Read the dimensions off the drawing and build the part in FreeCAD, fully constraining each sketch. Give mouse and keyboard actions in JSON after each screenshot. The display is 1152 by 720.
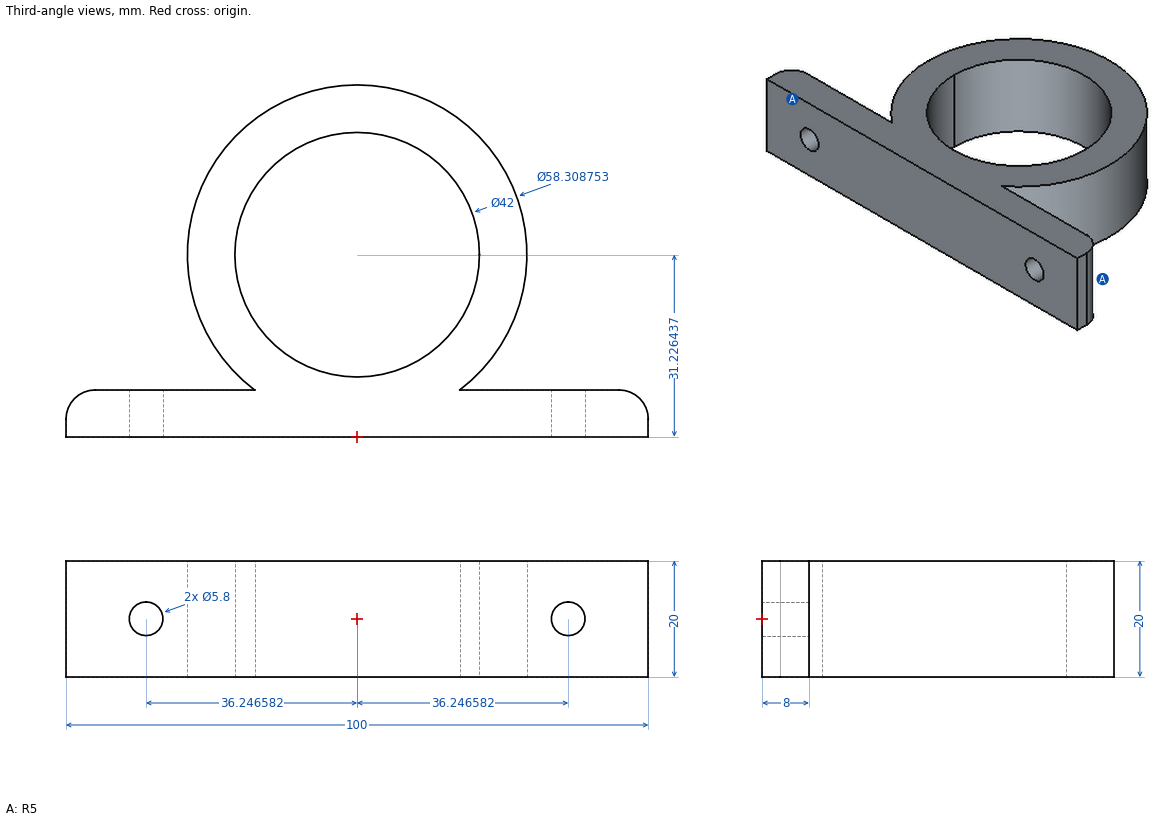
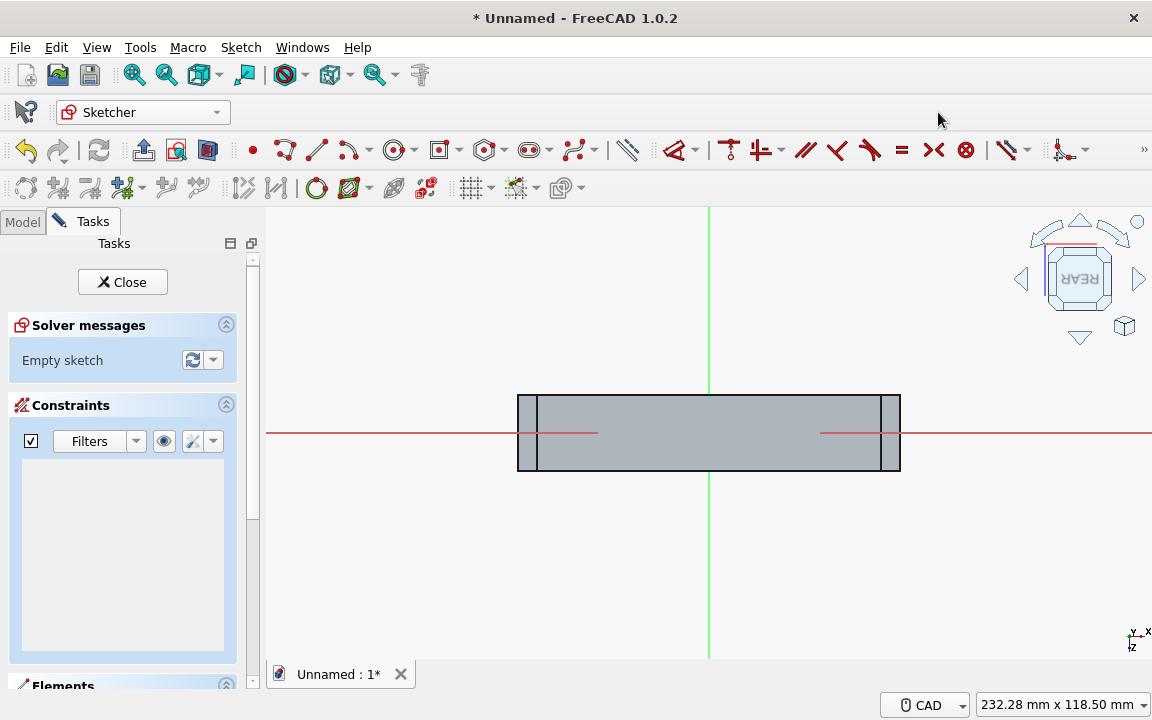
{"action": "scroll", "coordinate": [848, 433], "scroll_direction": "up", "scroll_amount": 2}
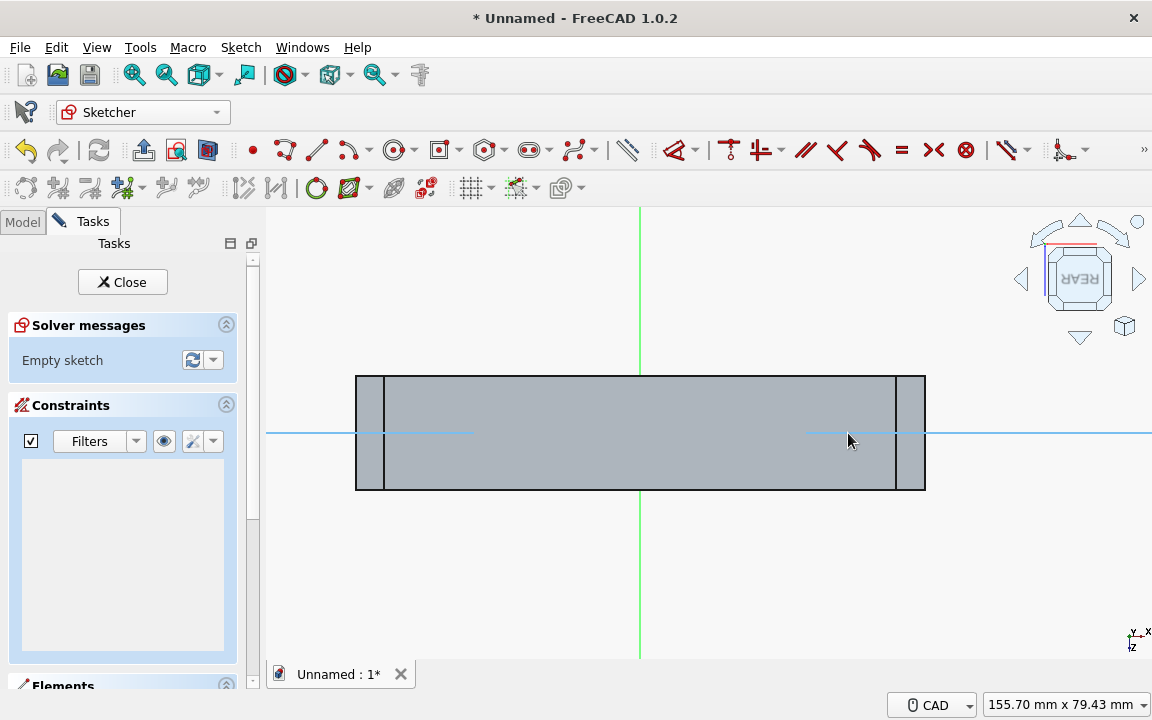
{"action": "left_click", "coordinate": [394, 150]}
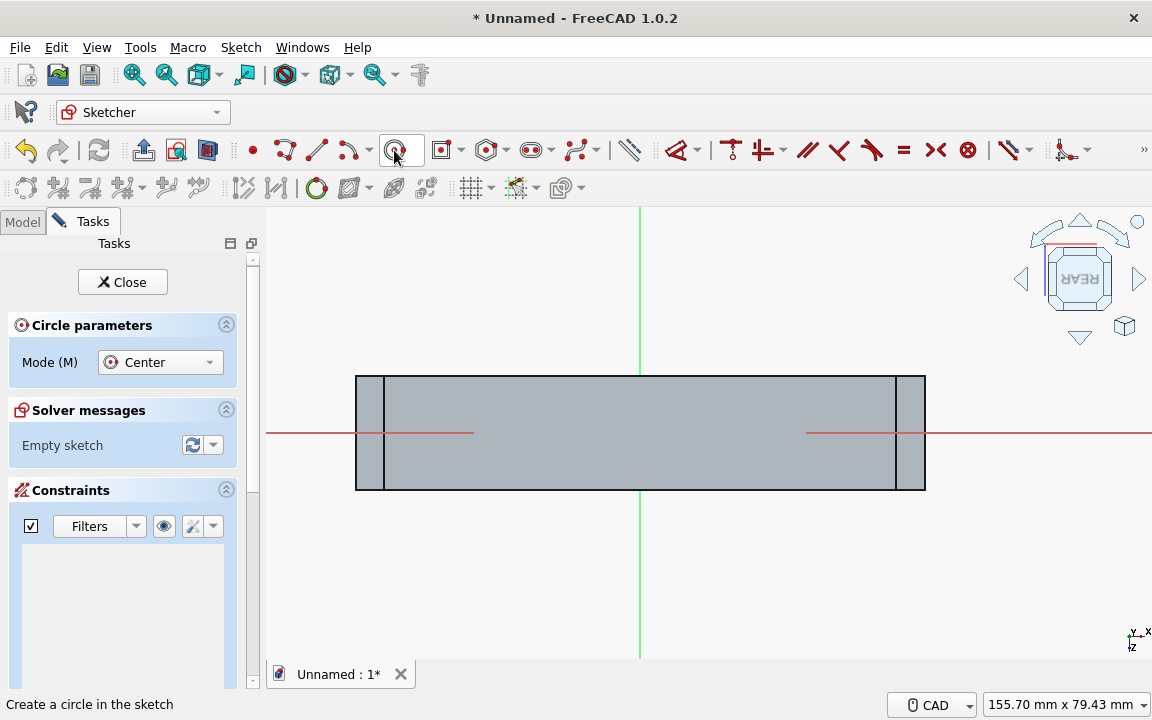
{"action": "scroll", "coordinate": [434, 433], "scroll_direction": "up", "scroll_amount": 2}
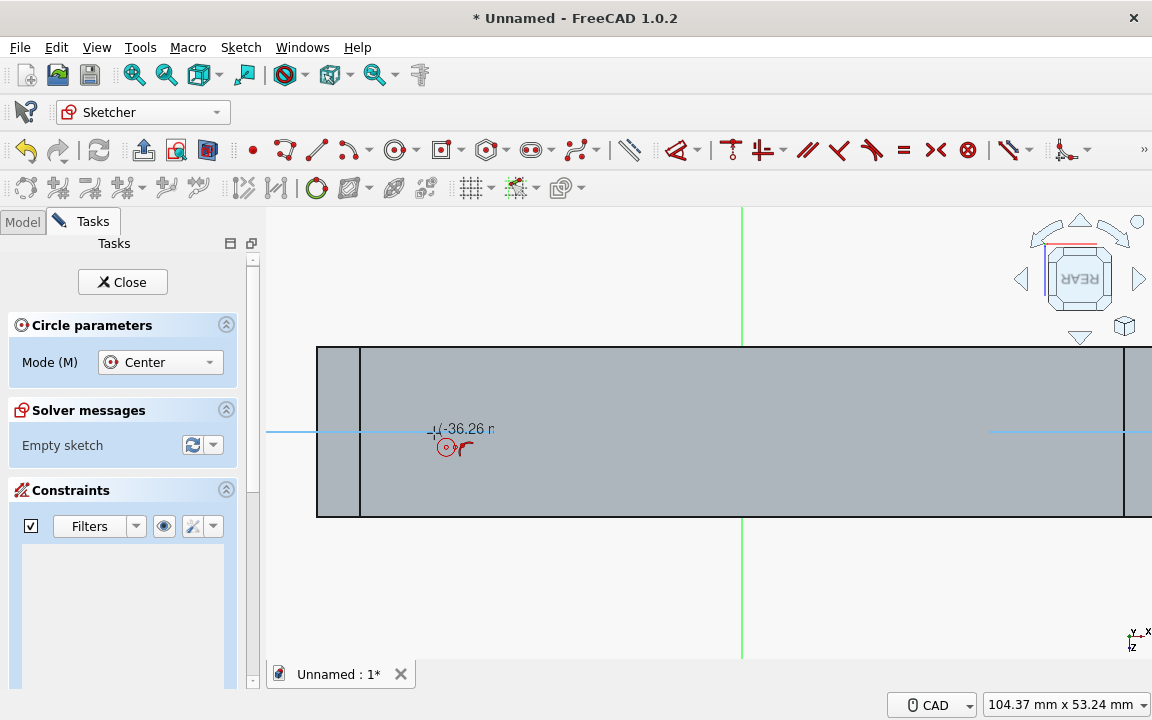
{"action": "left_click", "coordinate": [434, 432]}
{"action": "left_click", "coordinate": [451, 415]}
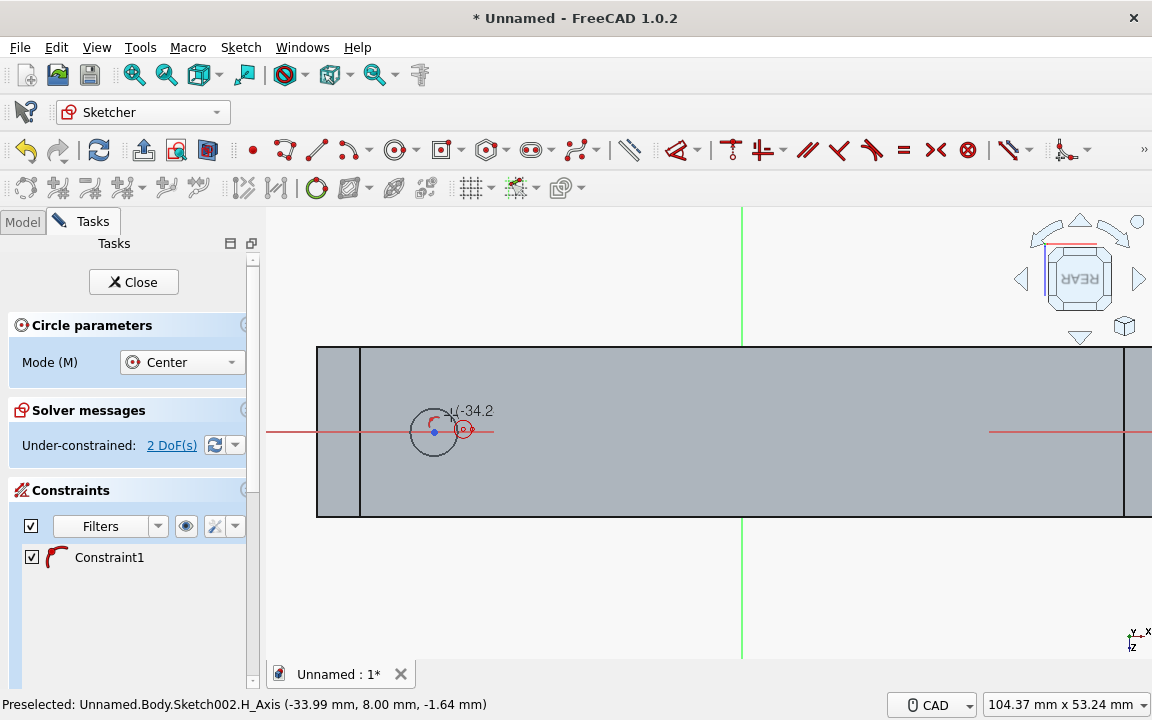
{"action": "scroll", "coordinate": [435, 434], "scroll_direction": "down", "scroll_amount": 2}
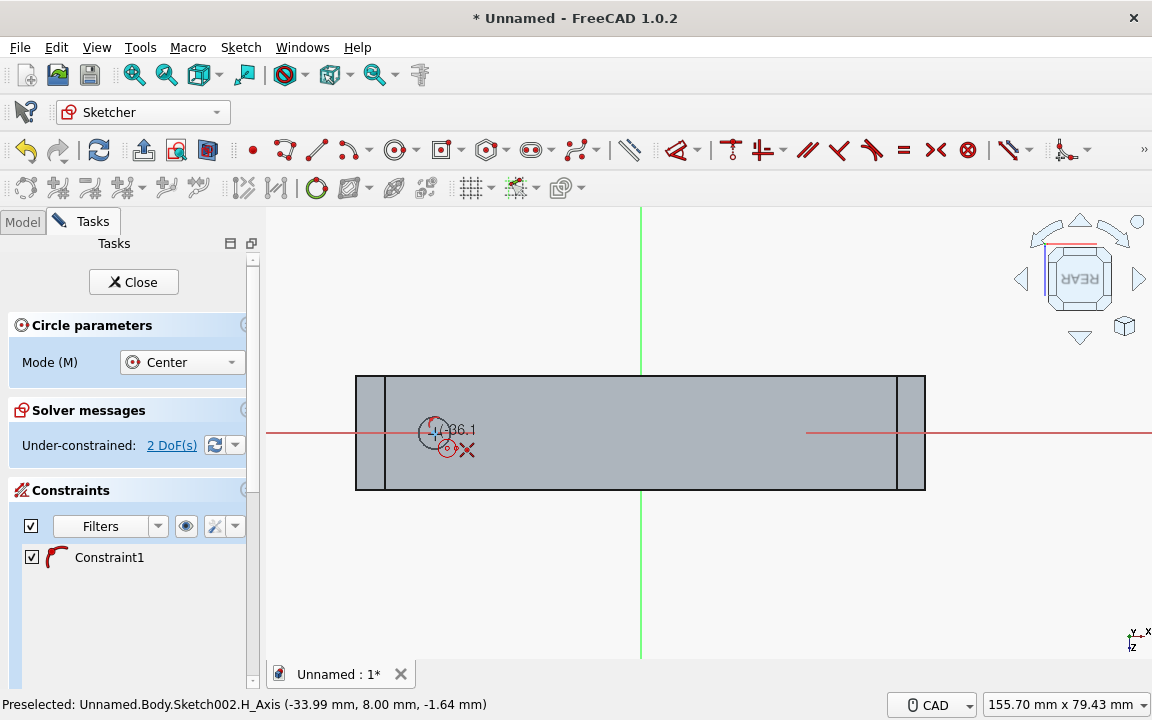
{"action": "scroll", "coordinate": [847, 433], "scroll_direction": "up", "scroll_amount": 2}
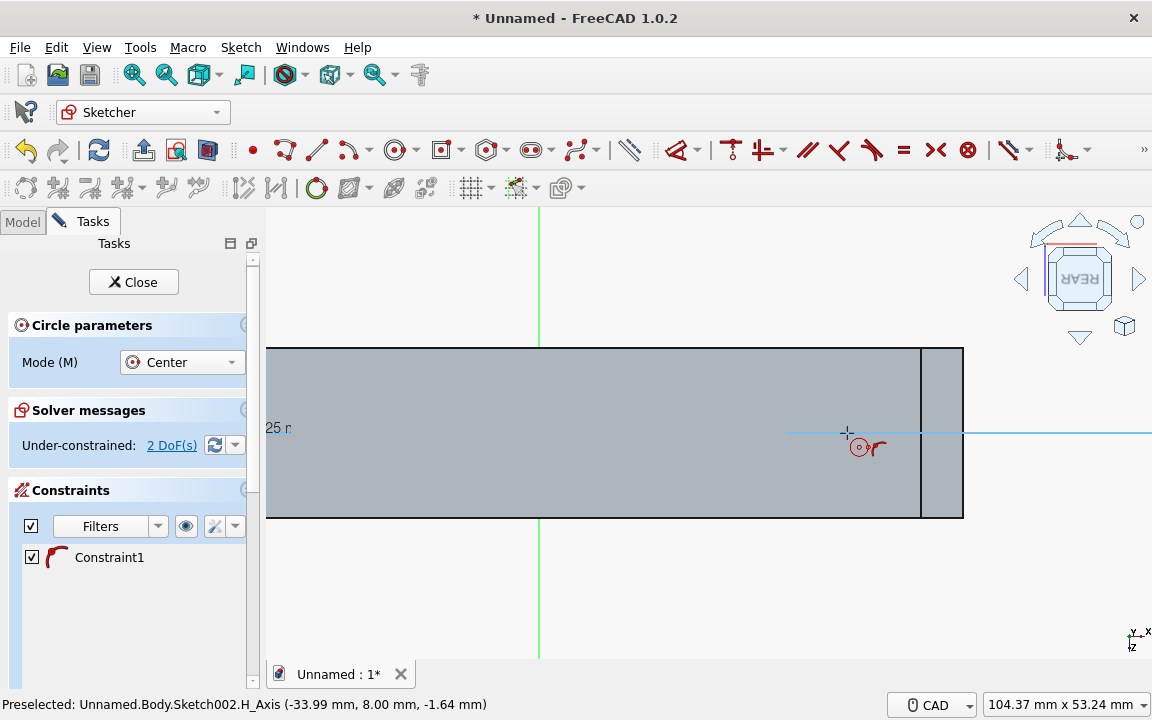
{"action": "left_click", "coordinate": [847, 433]}
{"action": "left_click", "coordinate": [864, 415]}
{"action": "key", "text": "Escape"}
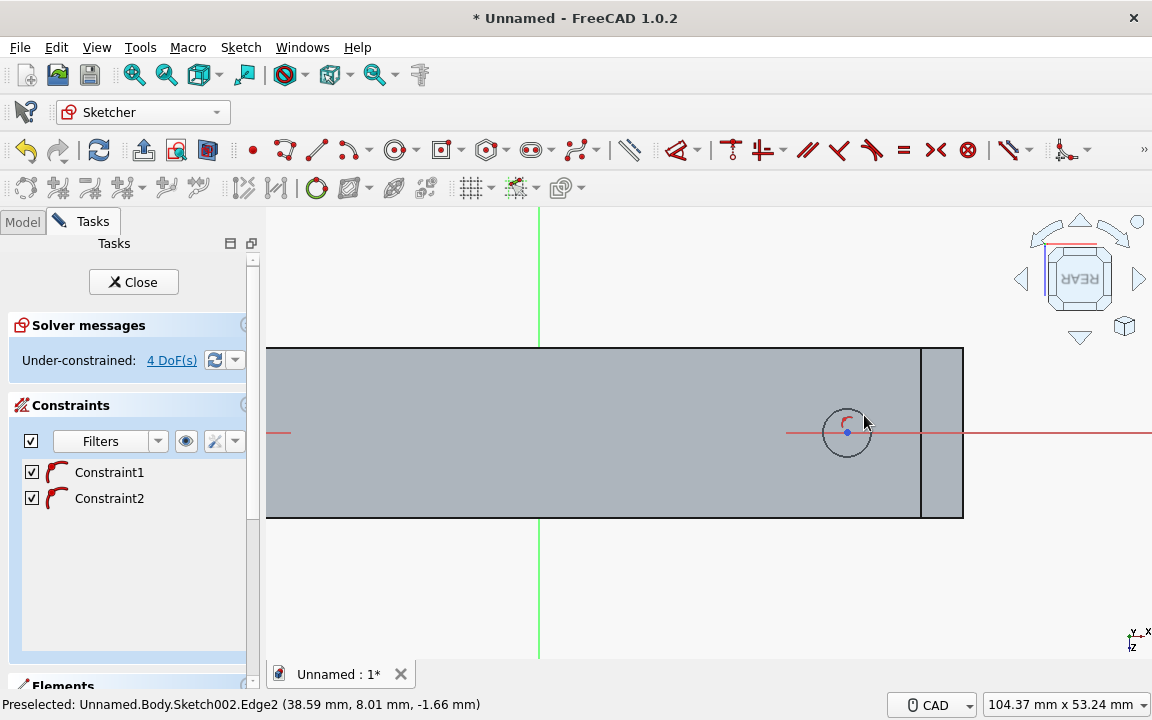
{"action": "scroll", "coordinate": [847, 433], "scroll_direction": "down", "scroll_amount": 2}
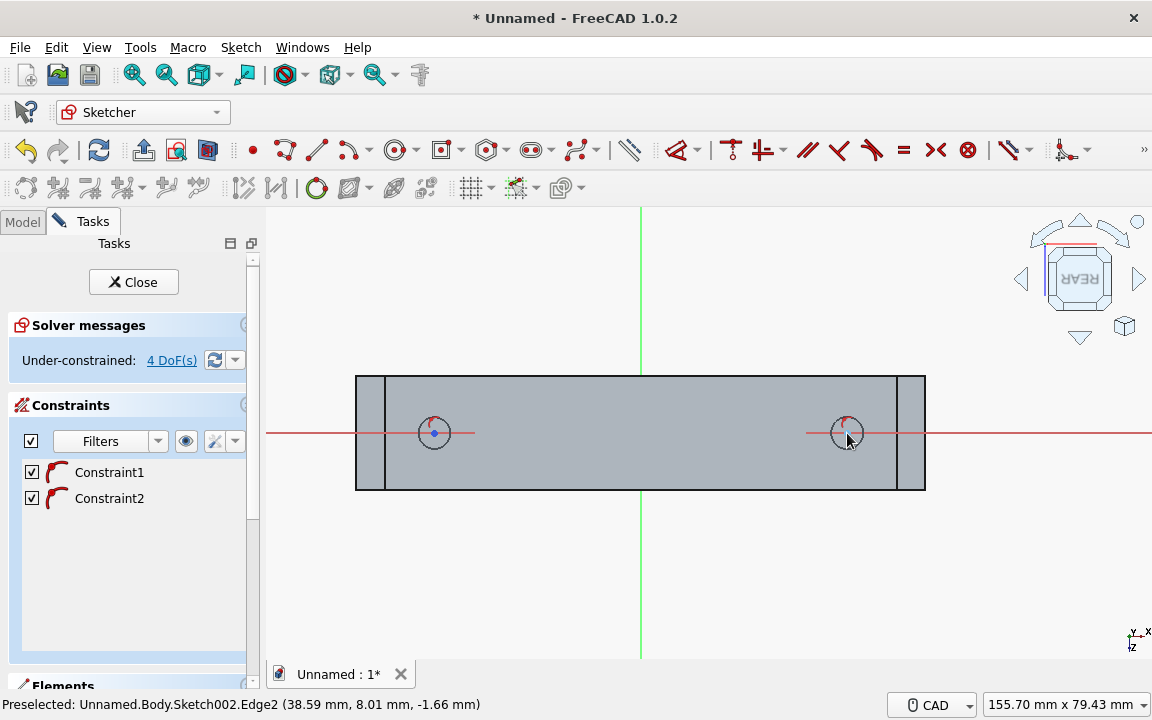
{"action": "scroll", "coordinate": [446, 422], "scroll_direction": "up", "scroll_amount": 2}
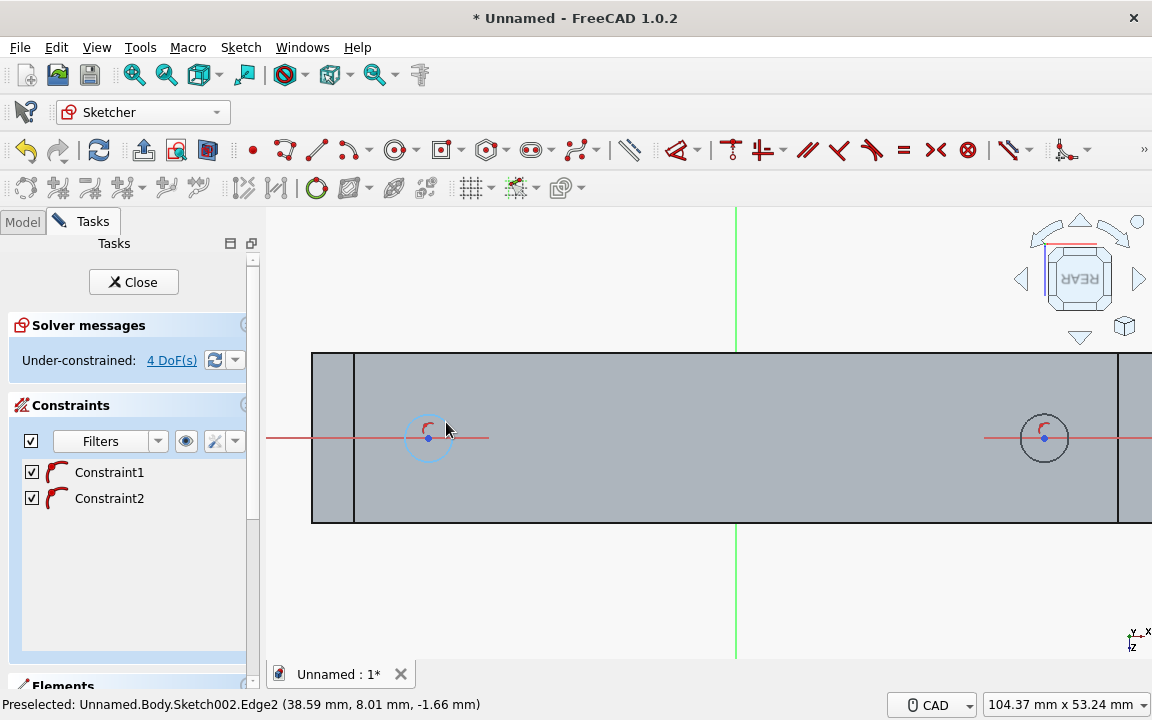
{"action": "left_click", "coordinate": [445, 422]}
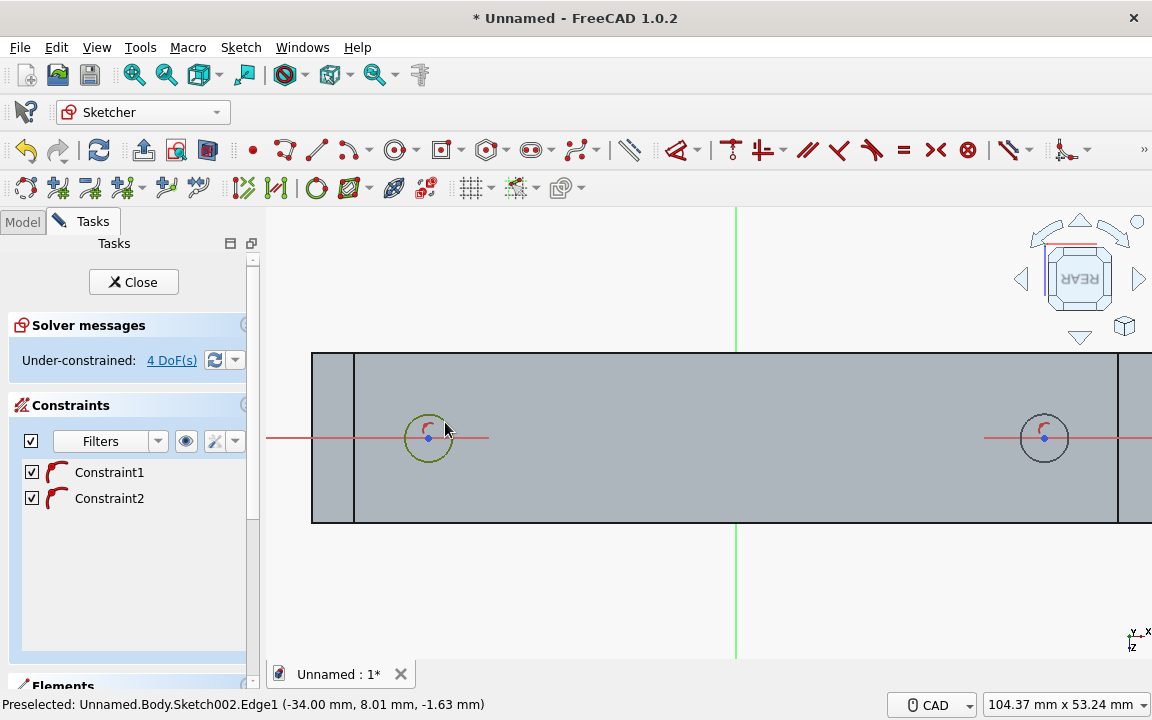
{"action": "scroll", "coordinate": [446, 422], "scroll_direction": "down", "scroll_amount": 2}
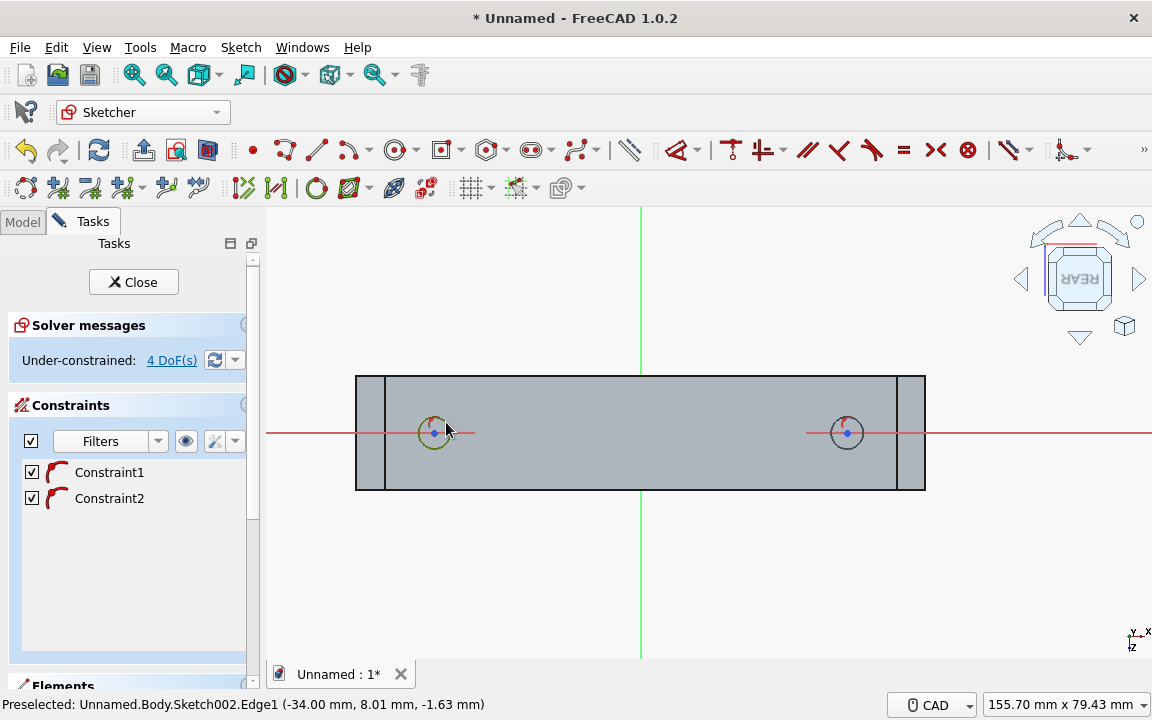
{"action": "left_click", "coordinate": [859, 422]}